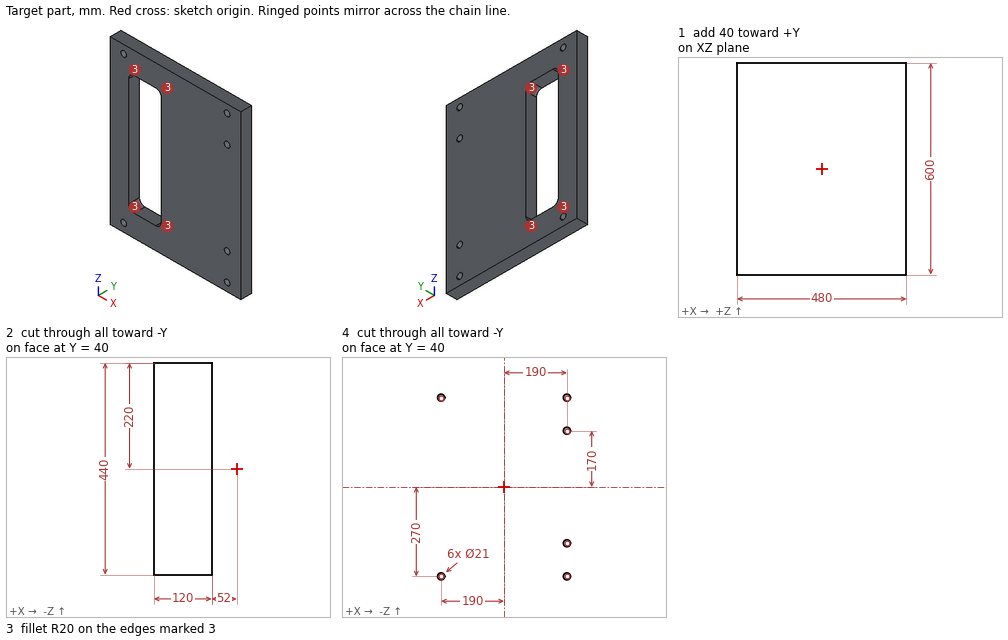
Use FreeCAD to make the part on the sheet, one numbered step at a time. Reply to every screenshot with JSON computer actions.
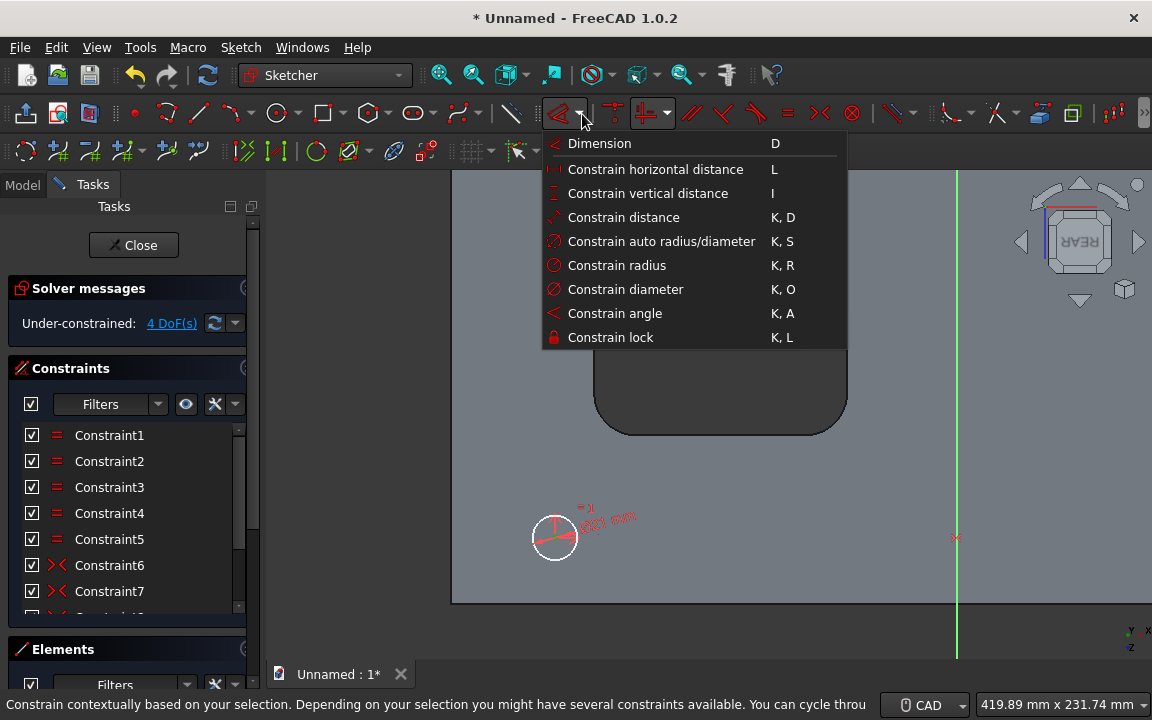
{"action": "left_click", "coordinate": [695, 169]}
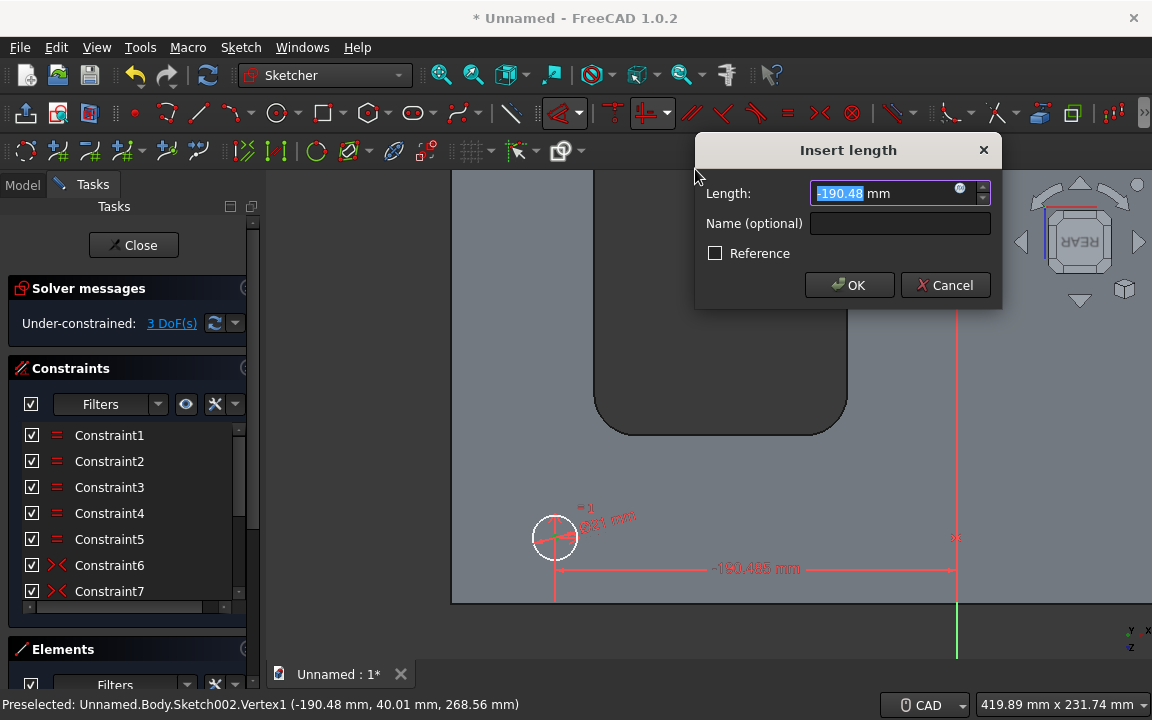
{"action": "type", "text": "-190"}
{"action": "key", "text": "Return"}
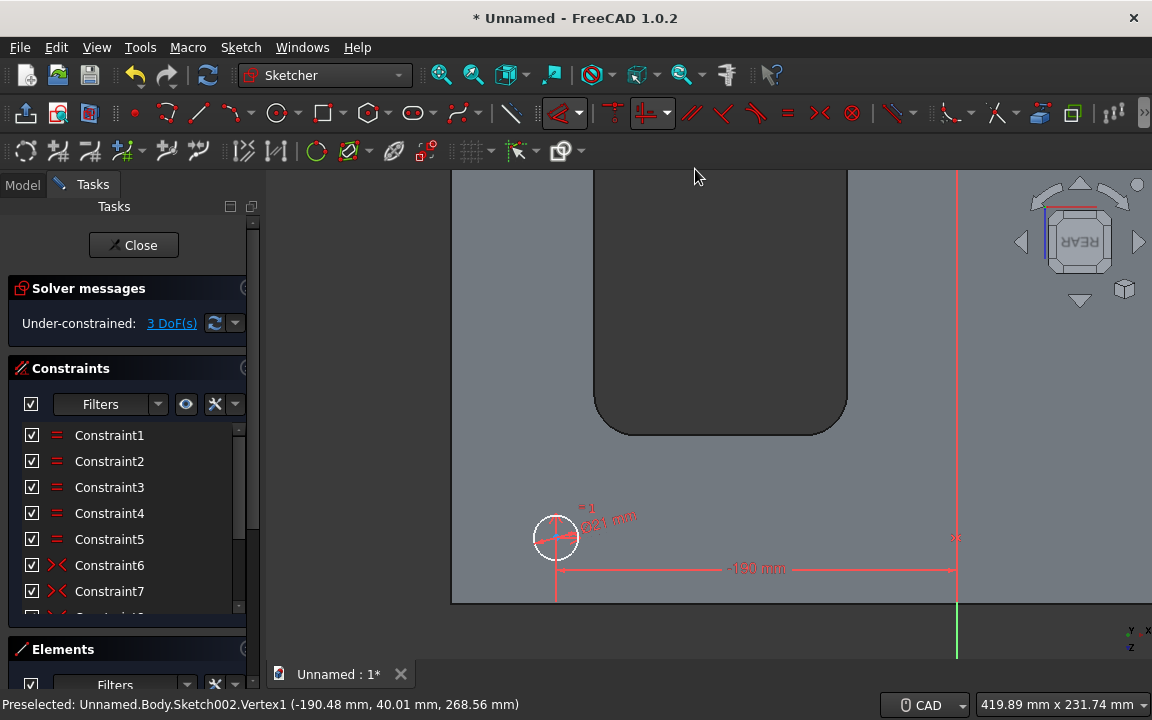
{"action": "left_click", "coordinate": [556, 538]}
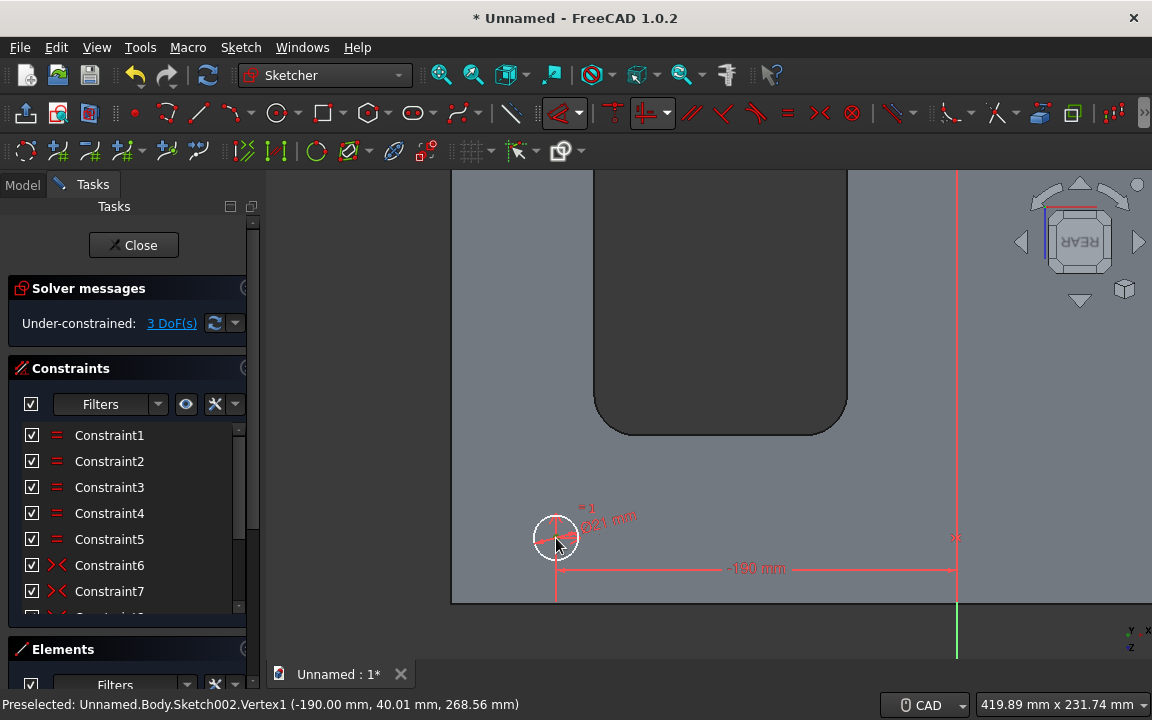
{"action": "left_click", "coordinate": [582, 114]}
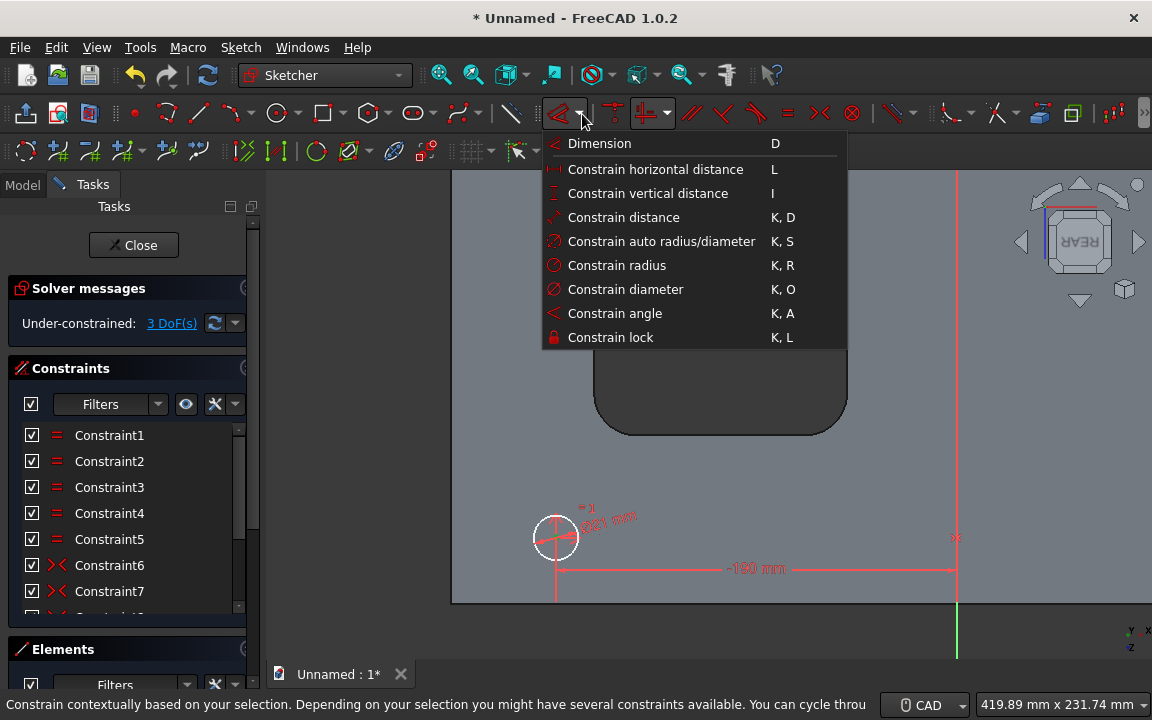
{"action": "left_click", "coordinate": [695, 193]}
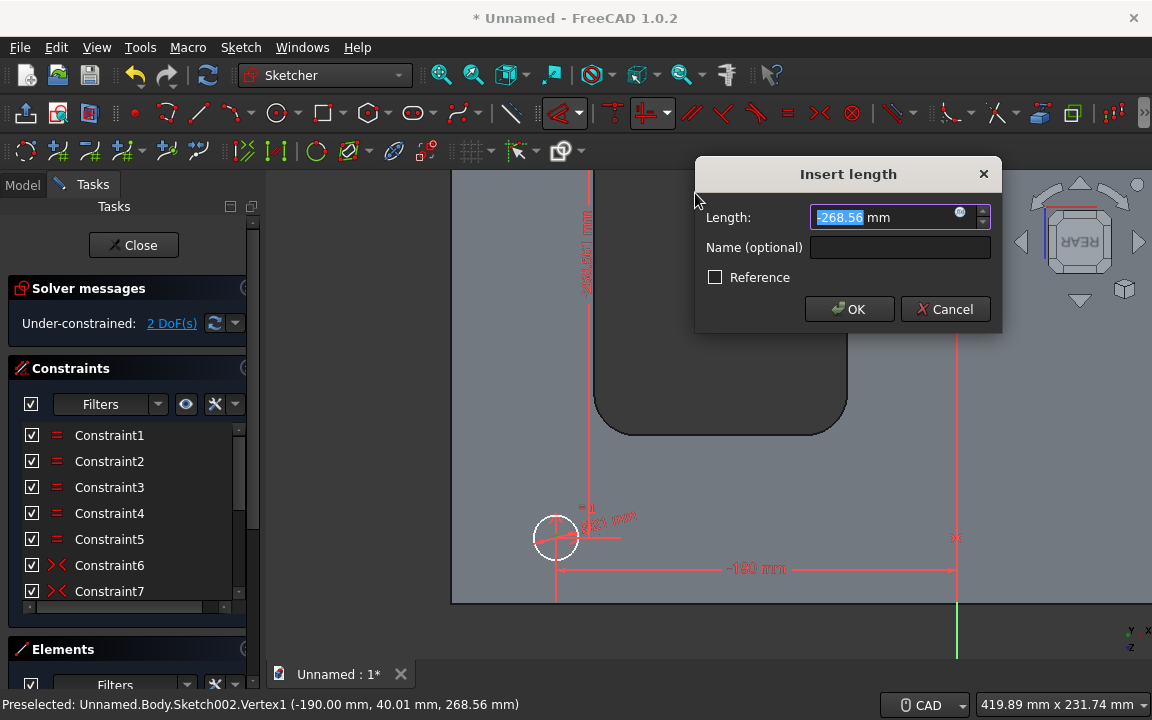
{"action": "type", "text": "-270"}
{"action": "key", "text": "Return"}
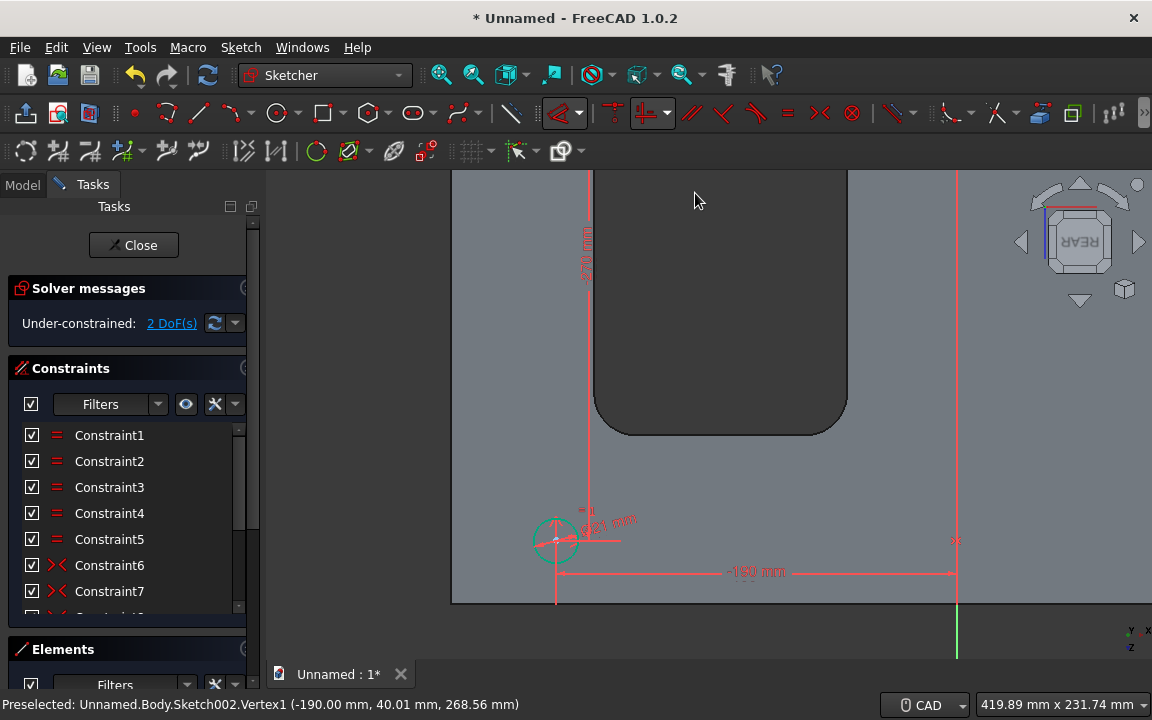
{"action": "scroll", "coordinate": [537, 560], "scroll_direction": "down", "scroll_amount": 7}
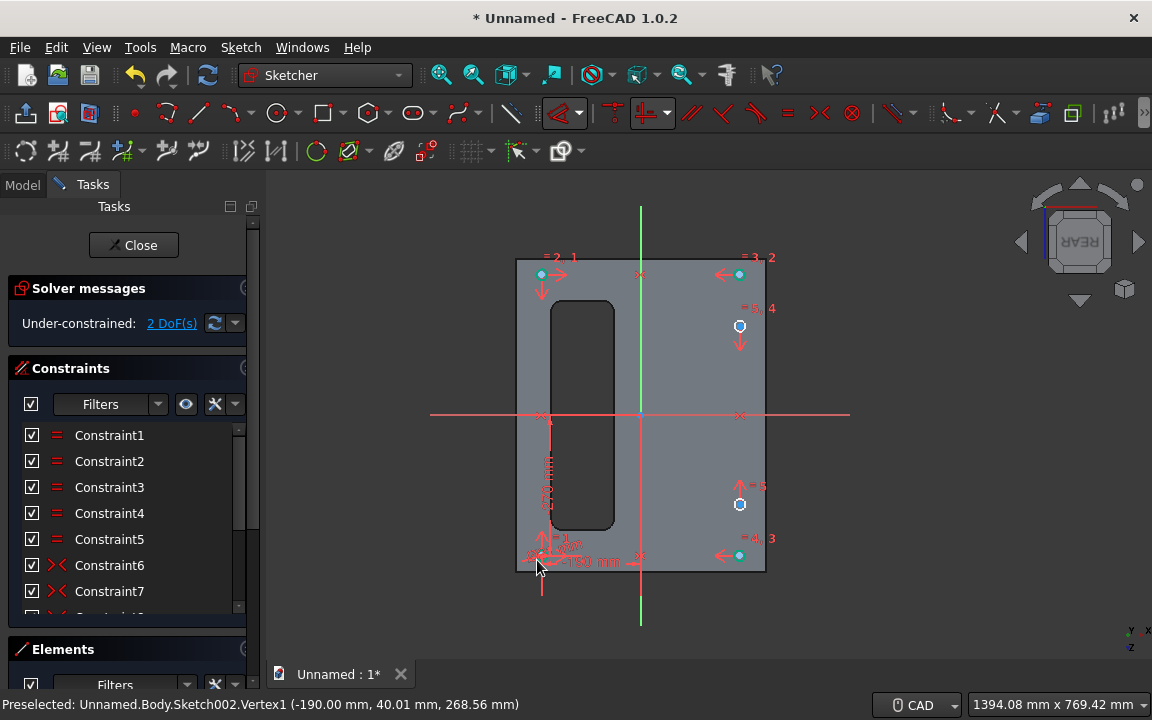
{"action": "left_click", "coordinate": [740, 326]}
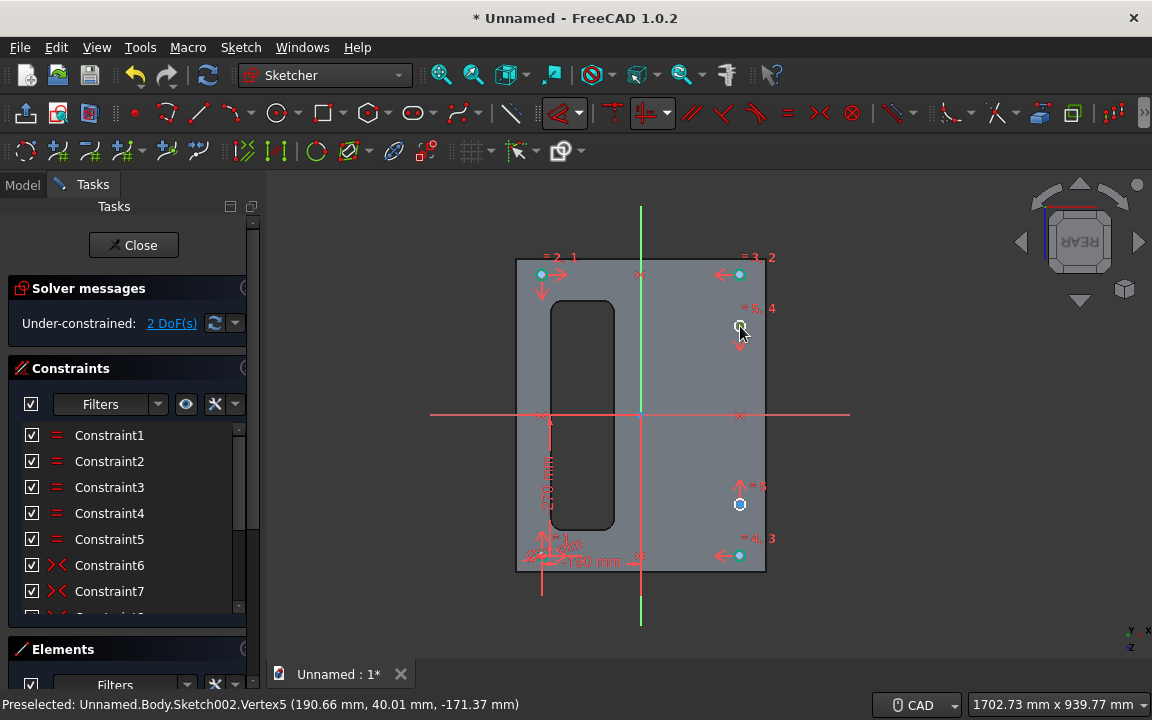
{"action": "left_click", "coordinate": [582, 114]}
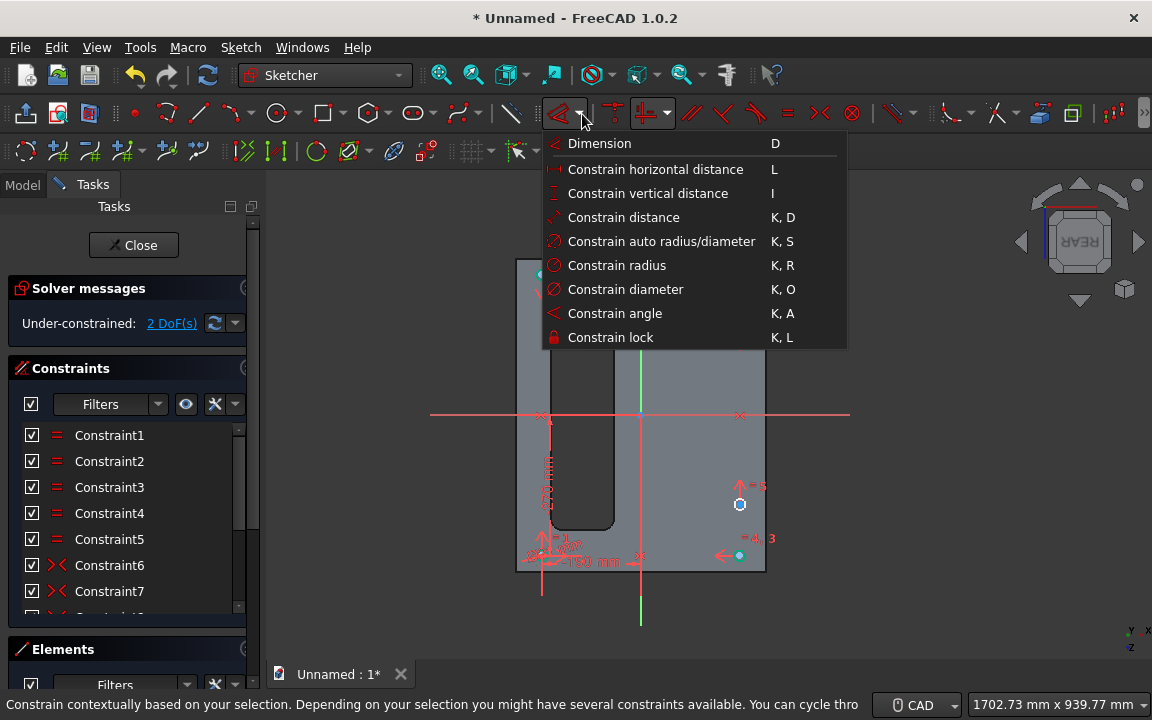
{"action": "left_click", "coordinate": [695, 169]}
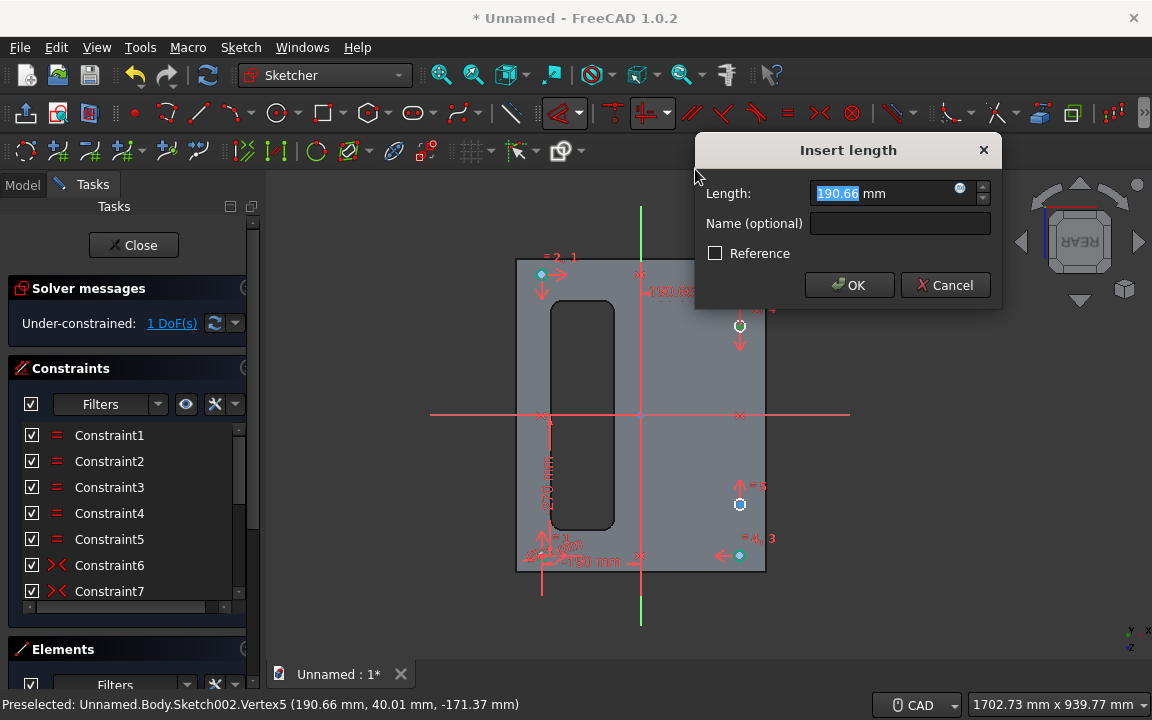
{"action": "type", "text": "190"}
{"action": "key", "text": "Return"}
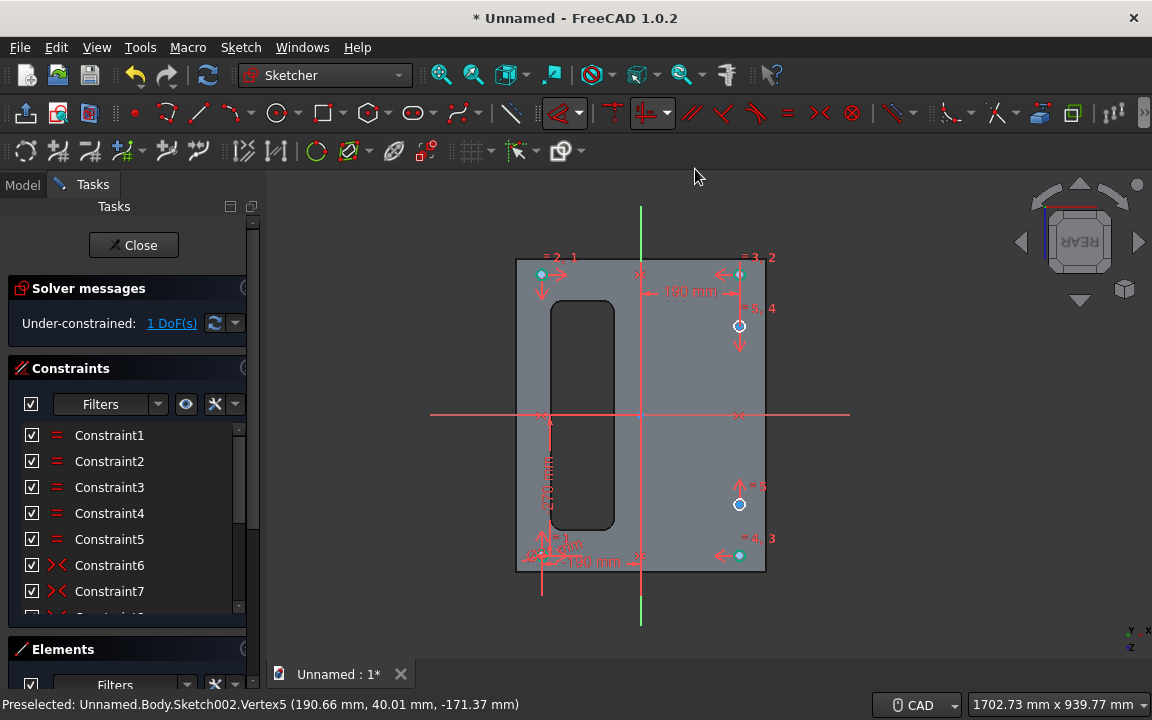
{"action": "left_click", "coordinate": [740, 326]}